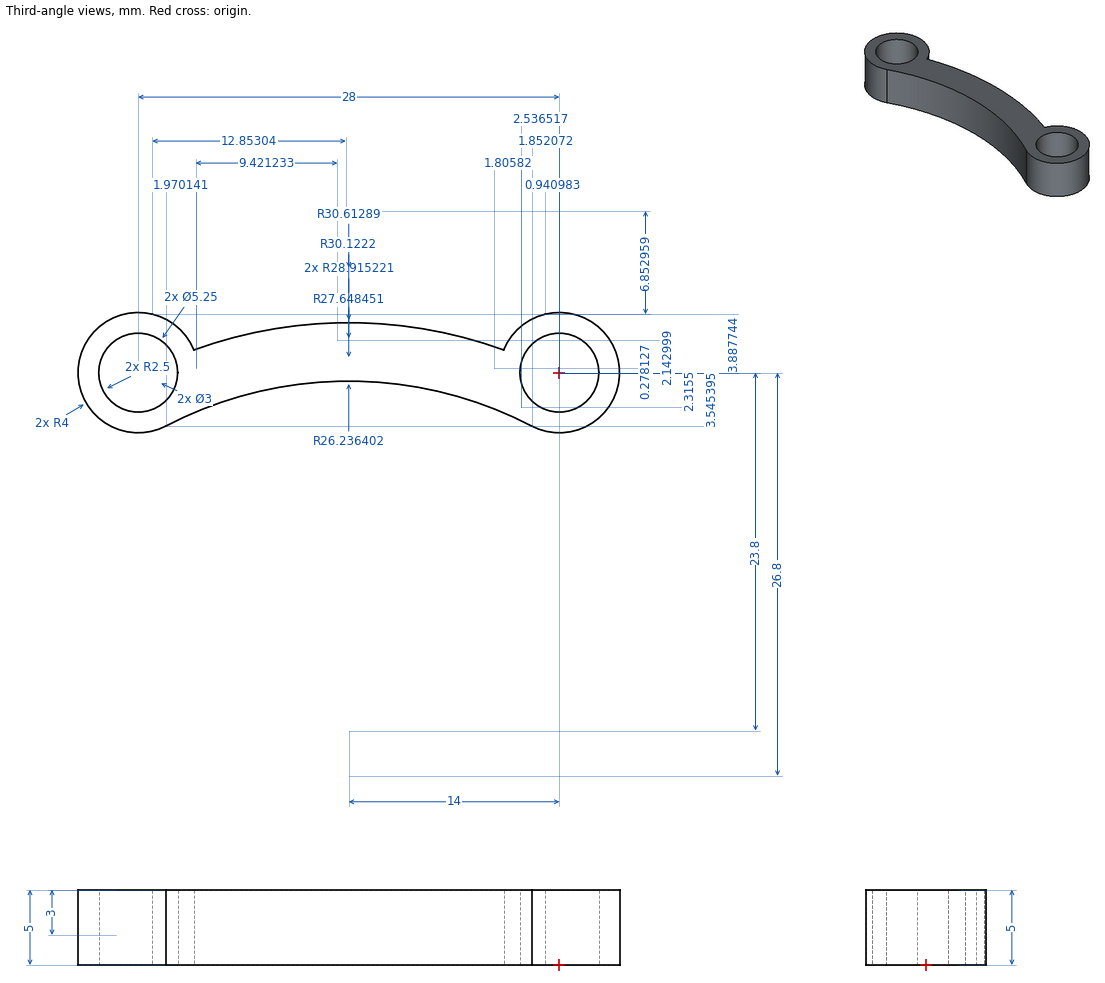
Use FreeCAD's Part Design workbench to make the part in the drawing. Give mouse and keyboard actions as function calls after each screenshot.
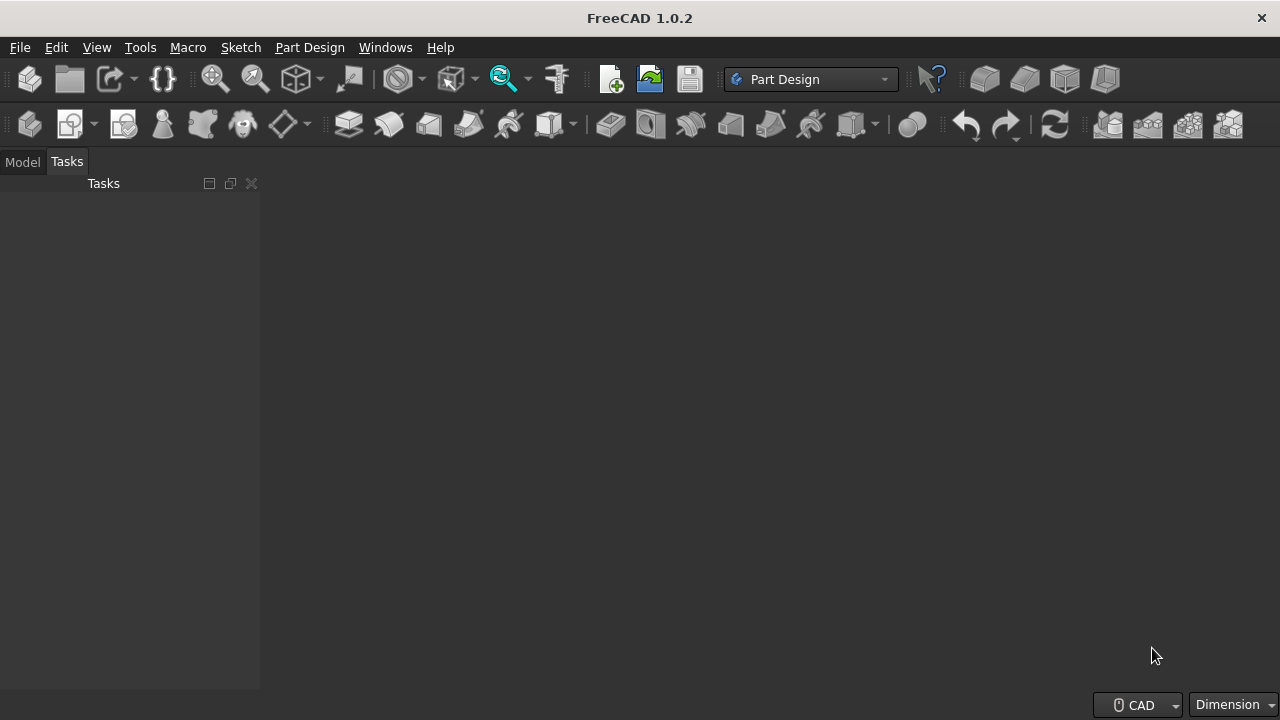
click(610, 80)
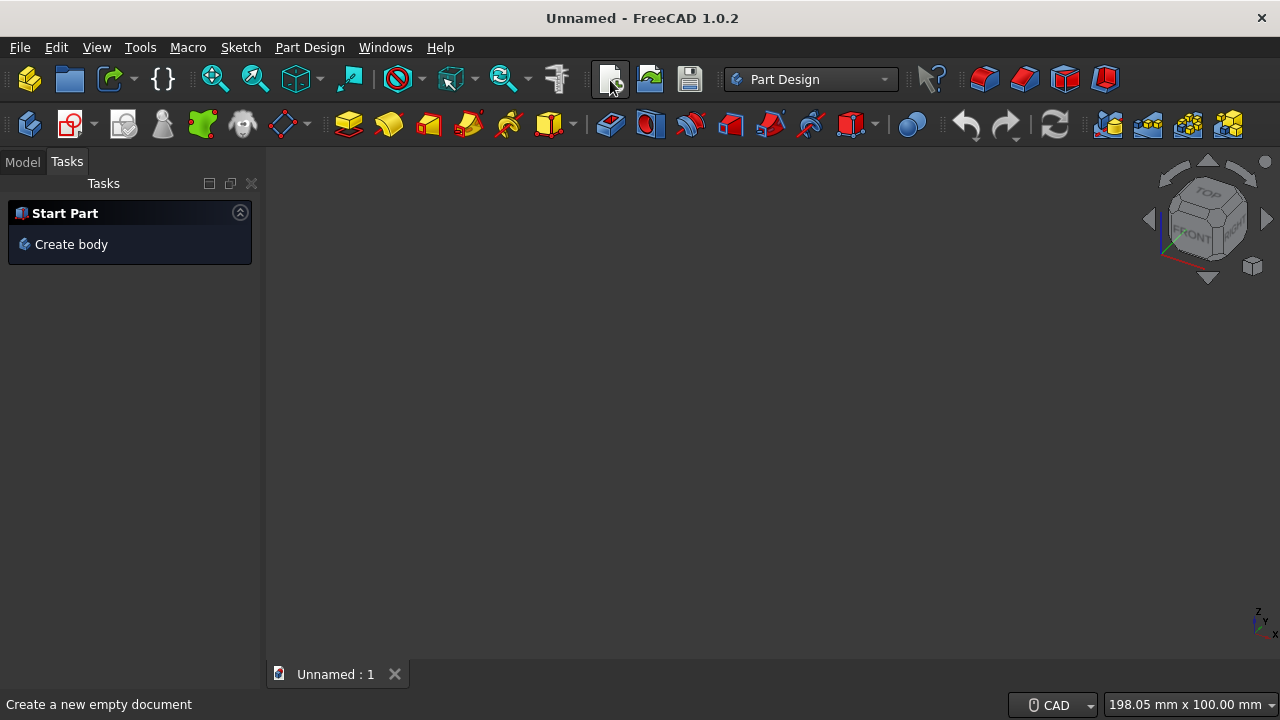
click(70, 124)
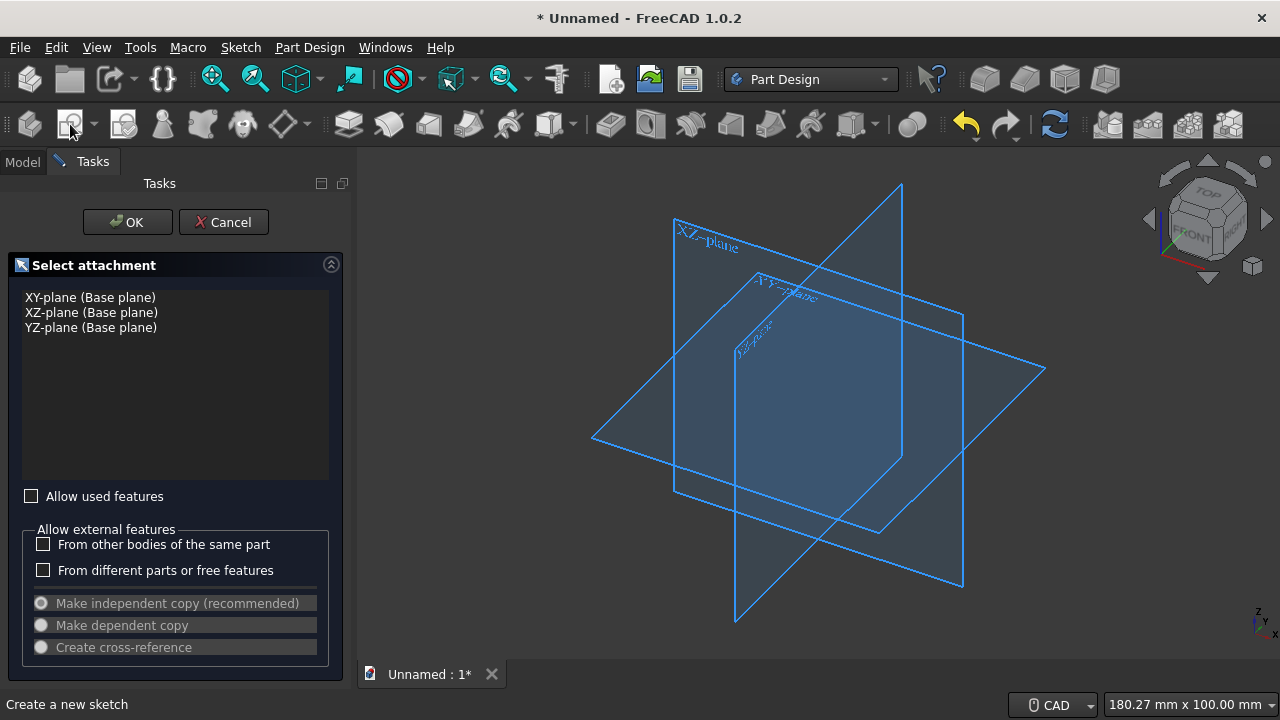
click(82, 298)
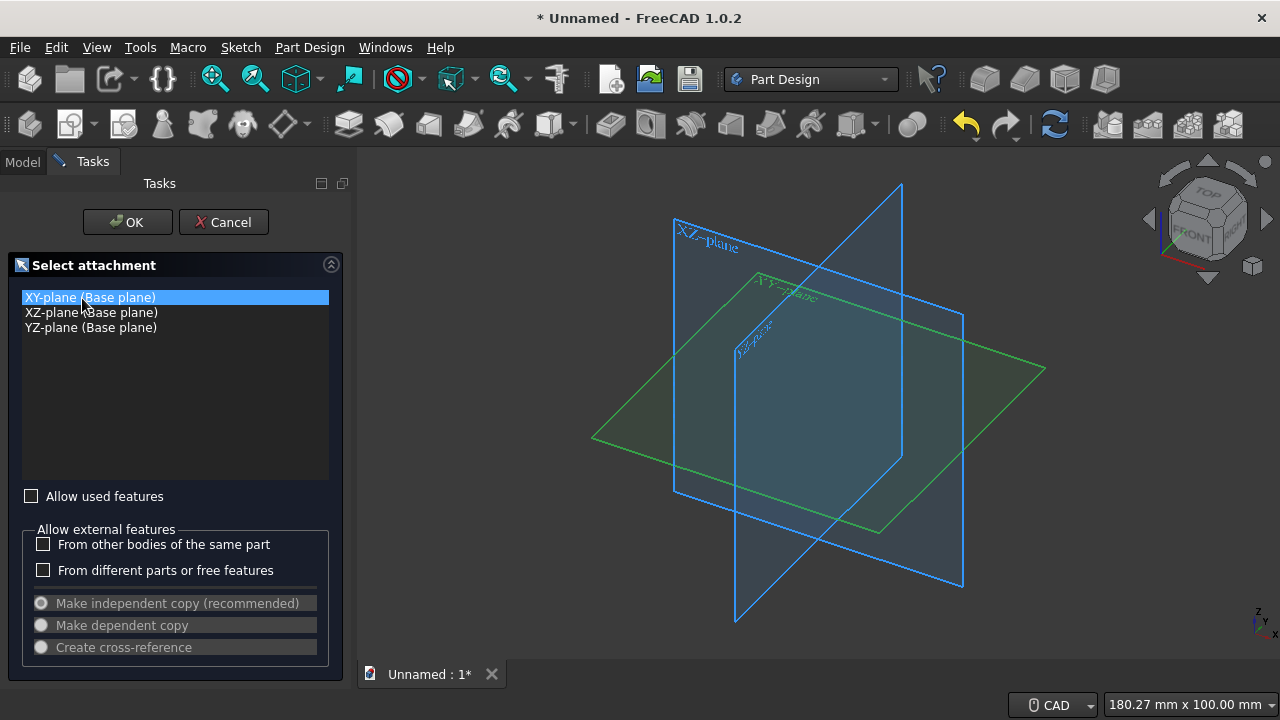
click(128, 222)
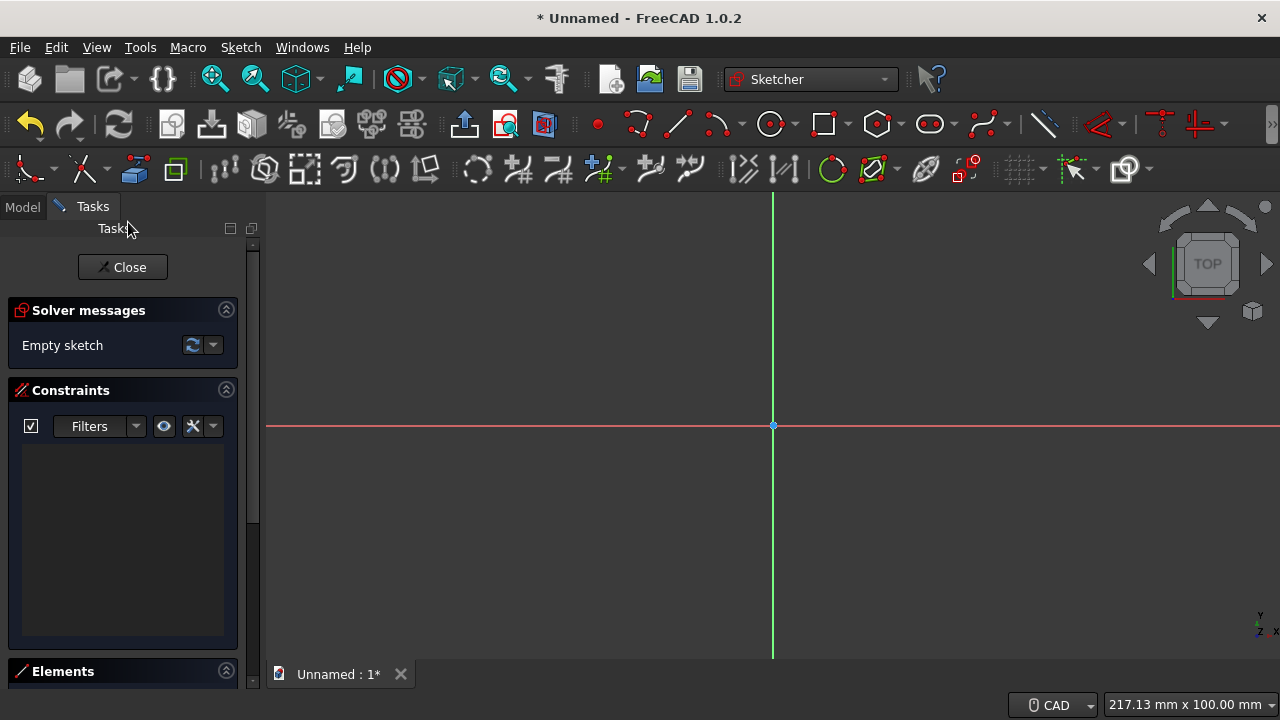
scroll(709, 413, up, 7)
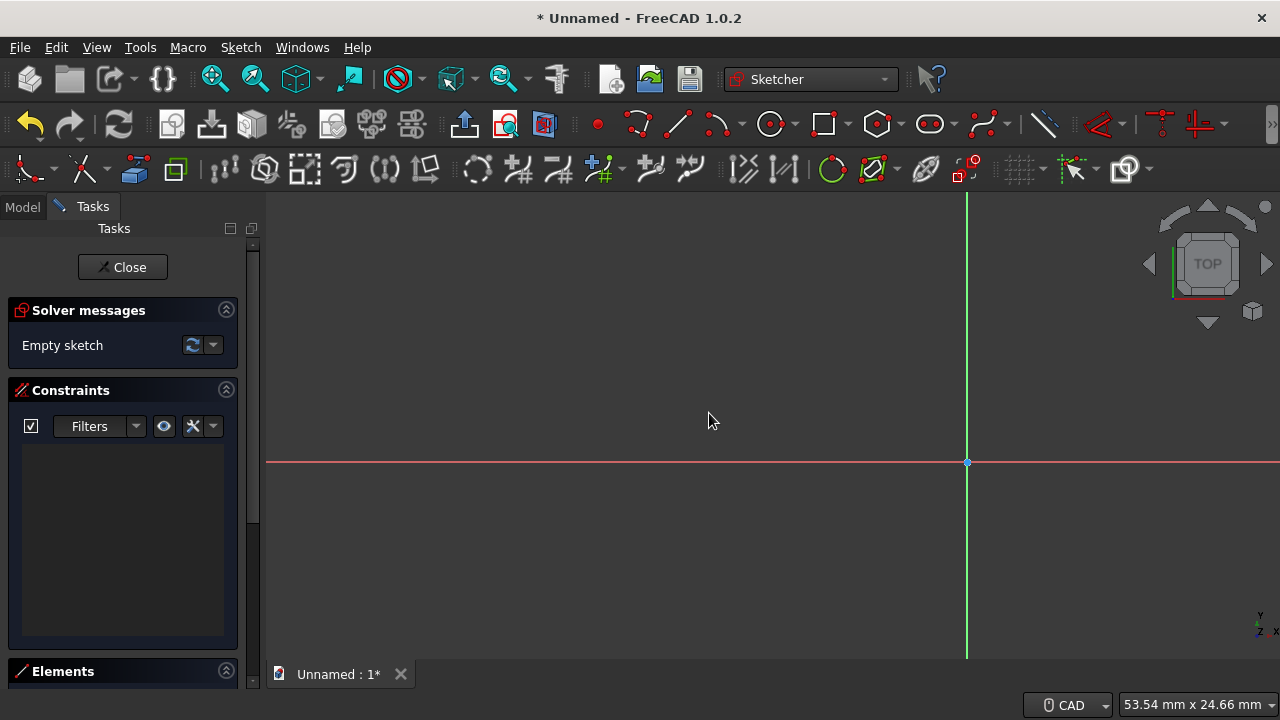
click(744, 124)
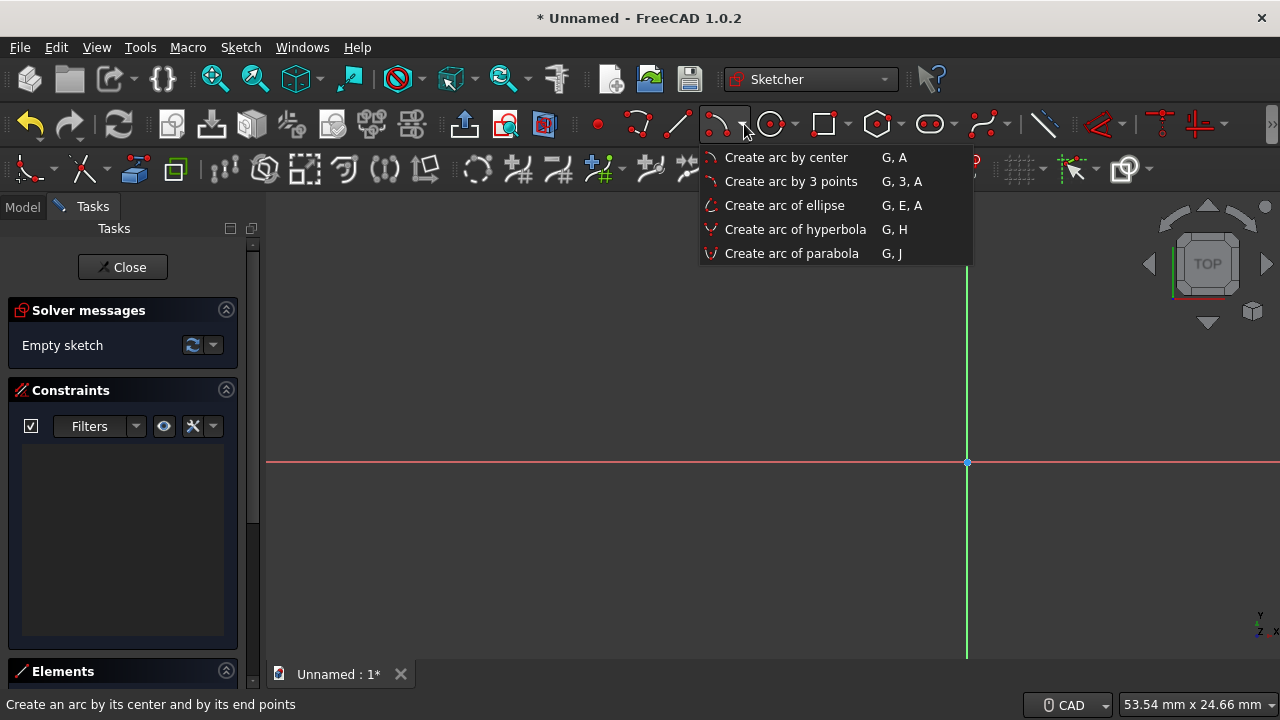
click(836, 181)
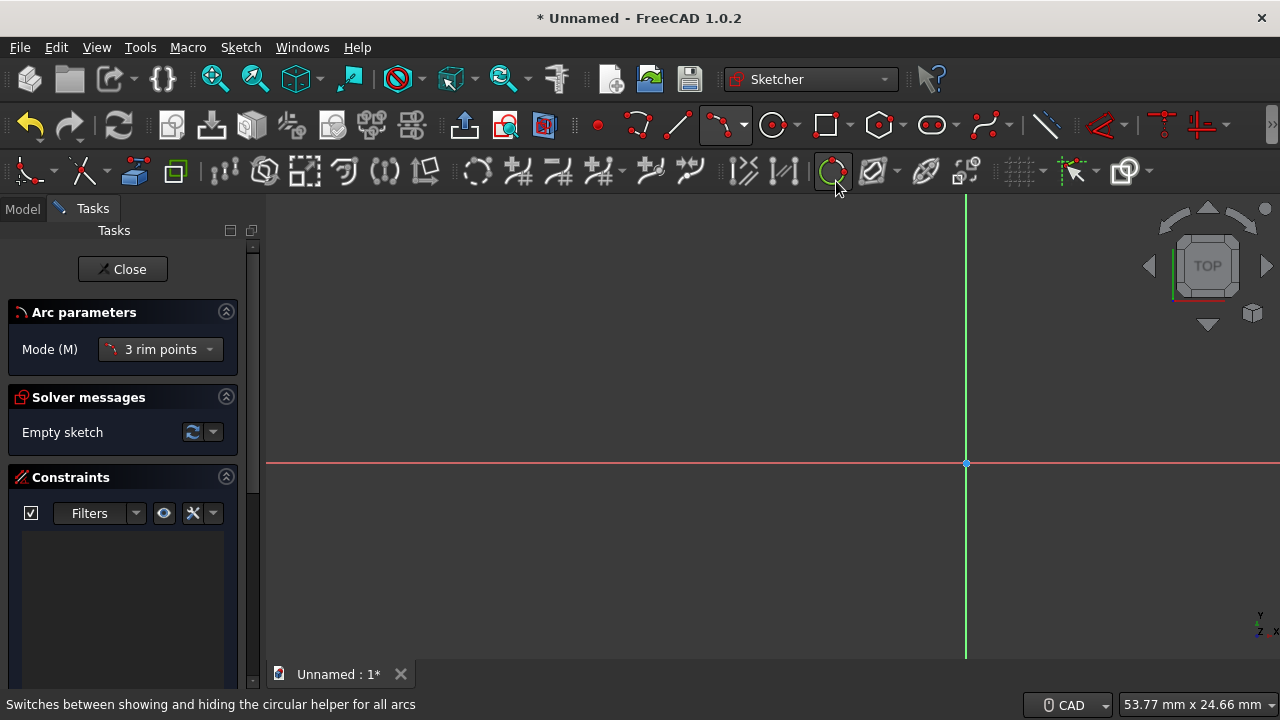
click(943, 422)
click(462, 422)
click(702, 367)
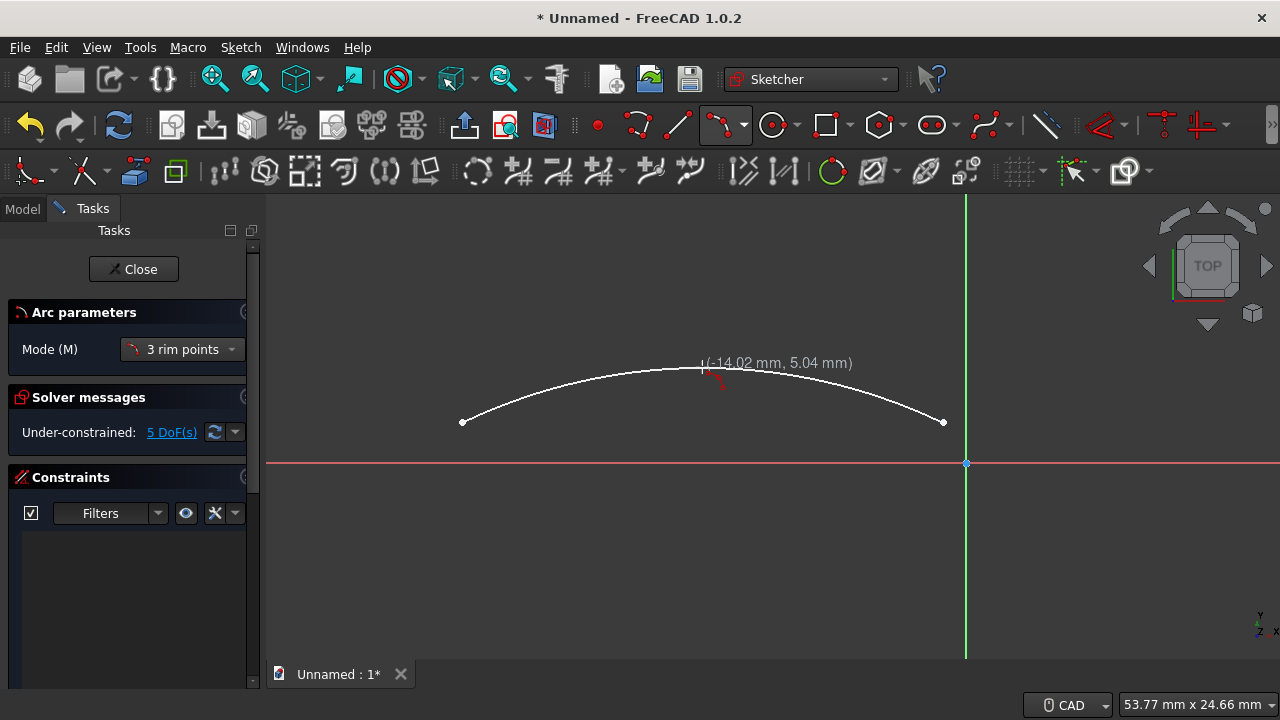
click(462, 423)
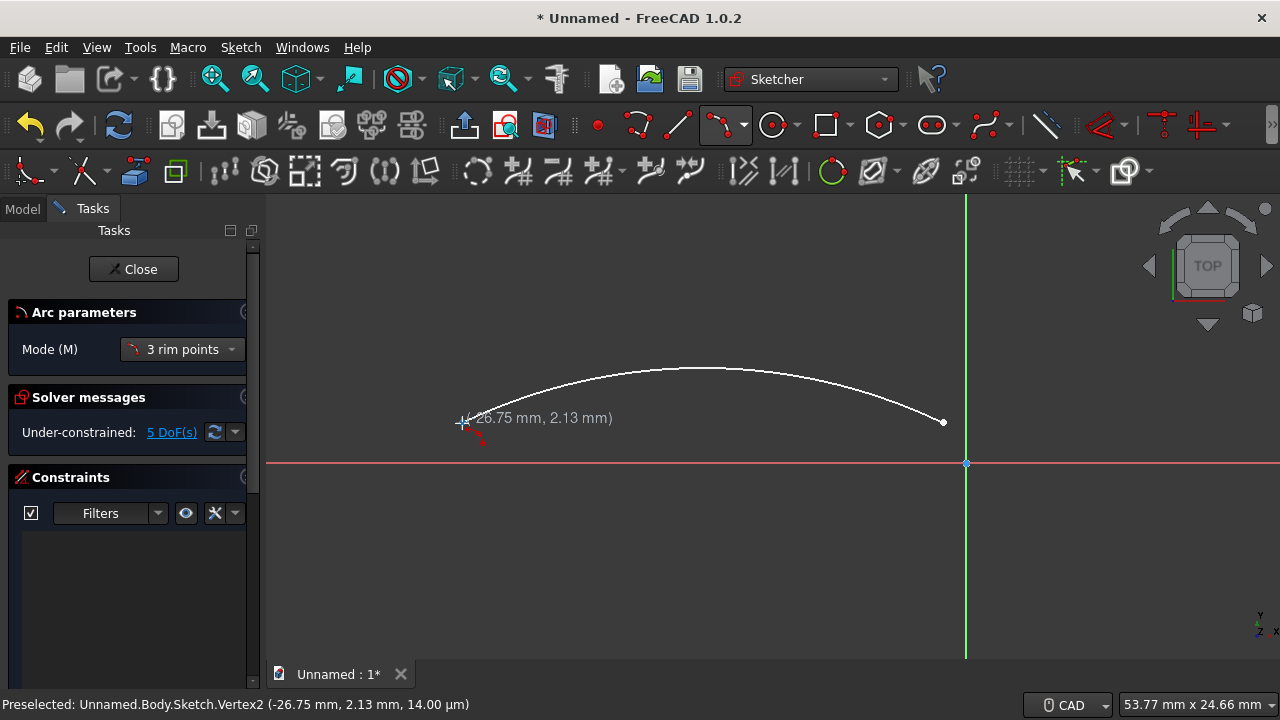
scroll(485, 468, up, 6)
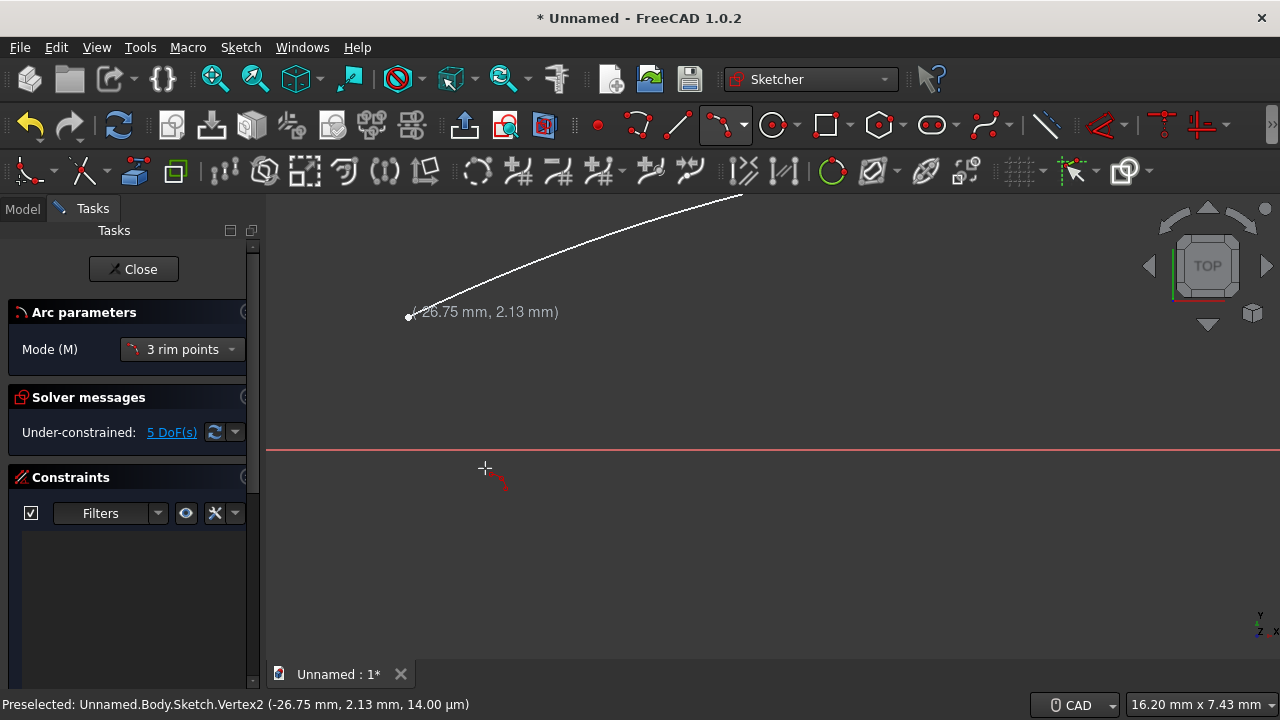
click(485, 468)